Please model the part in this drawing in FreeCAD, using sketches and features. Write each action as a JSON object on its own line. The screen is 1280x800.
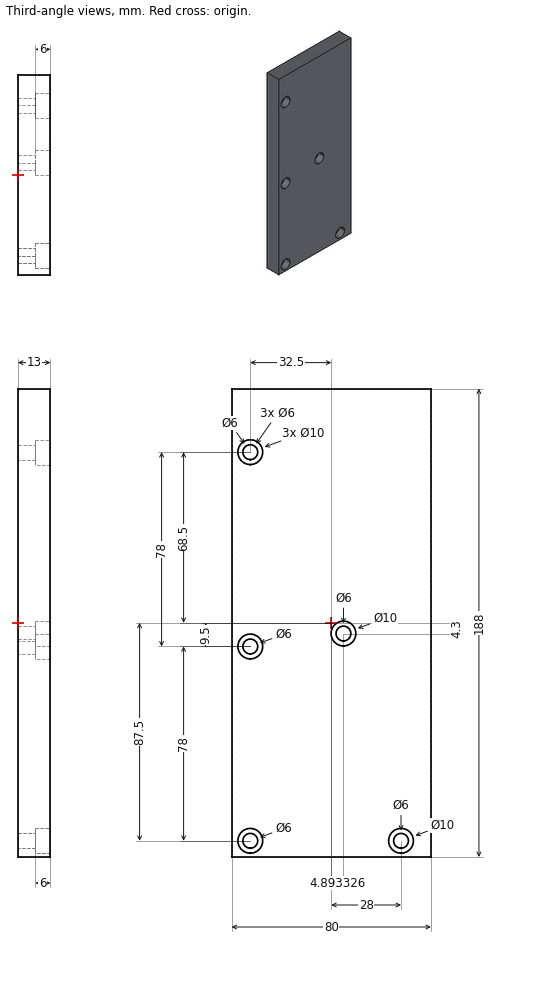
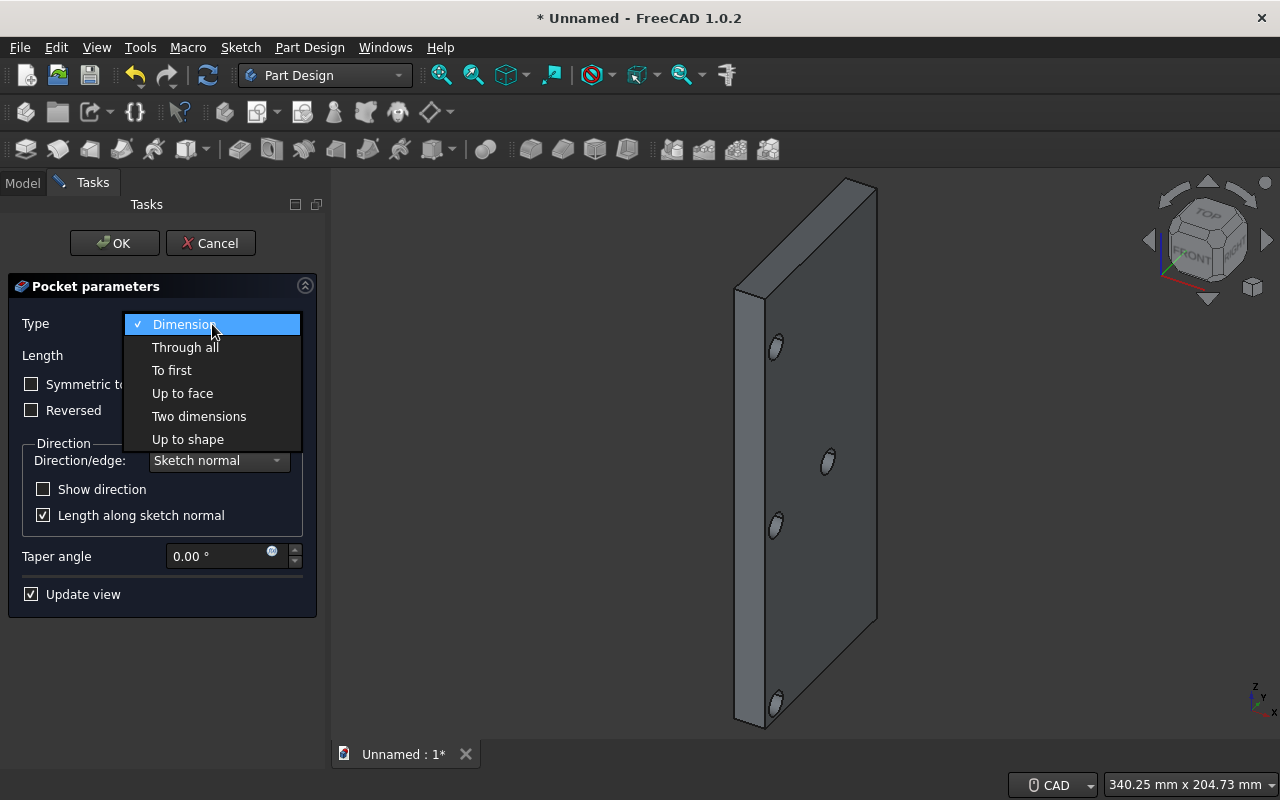
{"action": "left_click", "coordinate": [212, 370]}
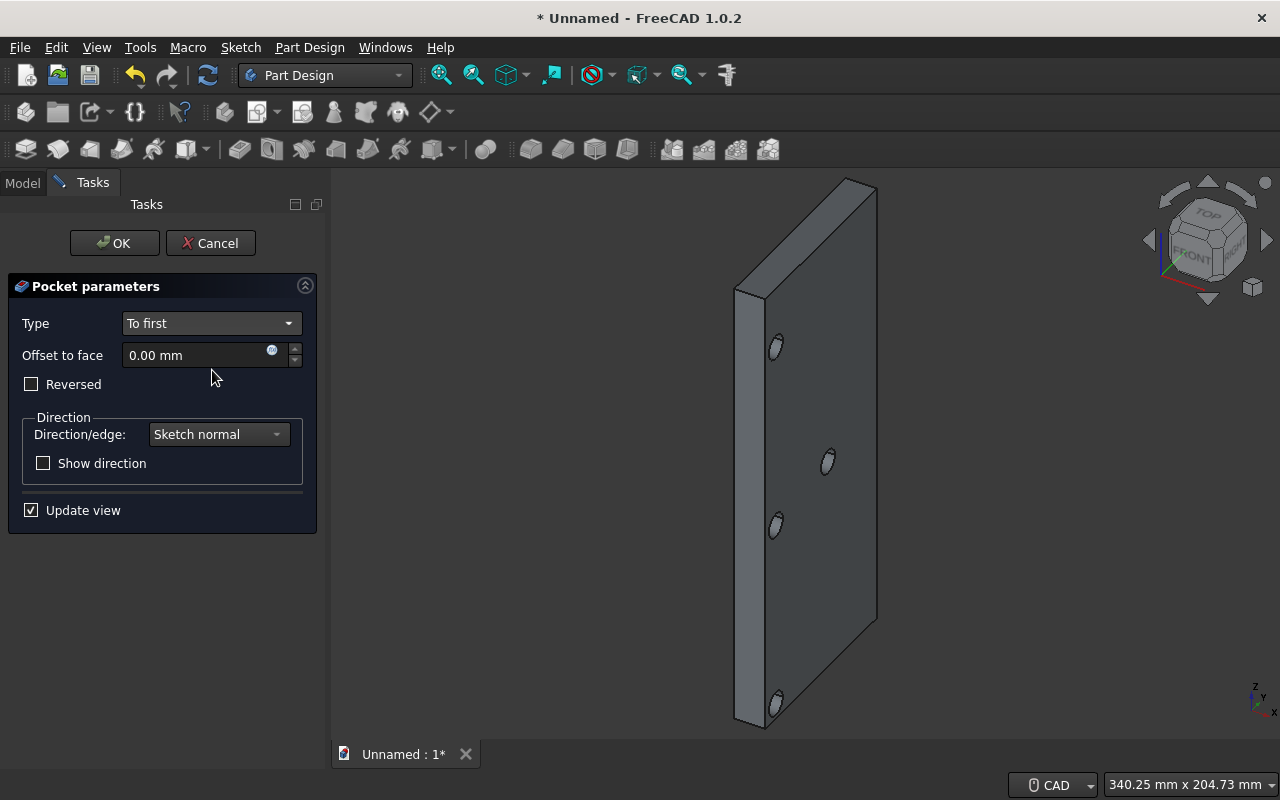
{"action": "left_click", "coordinate": [115, 243]}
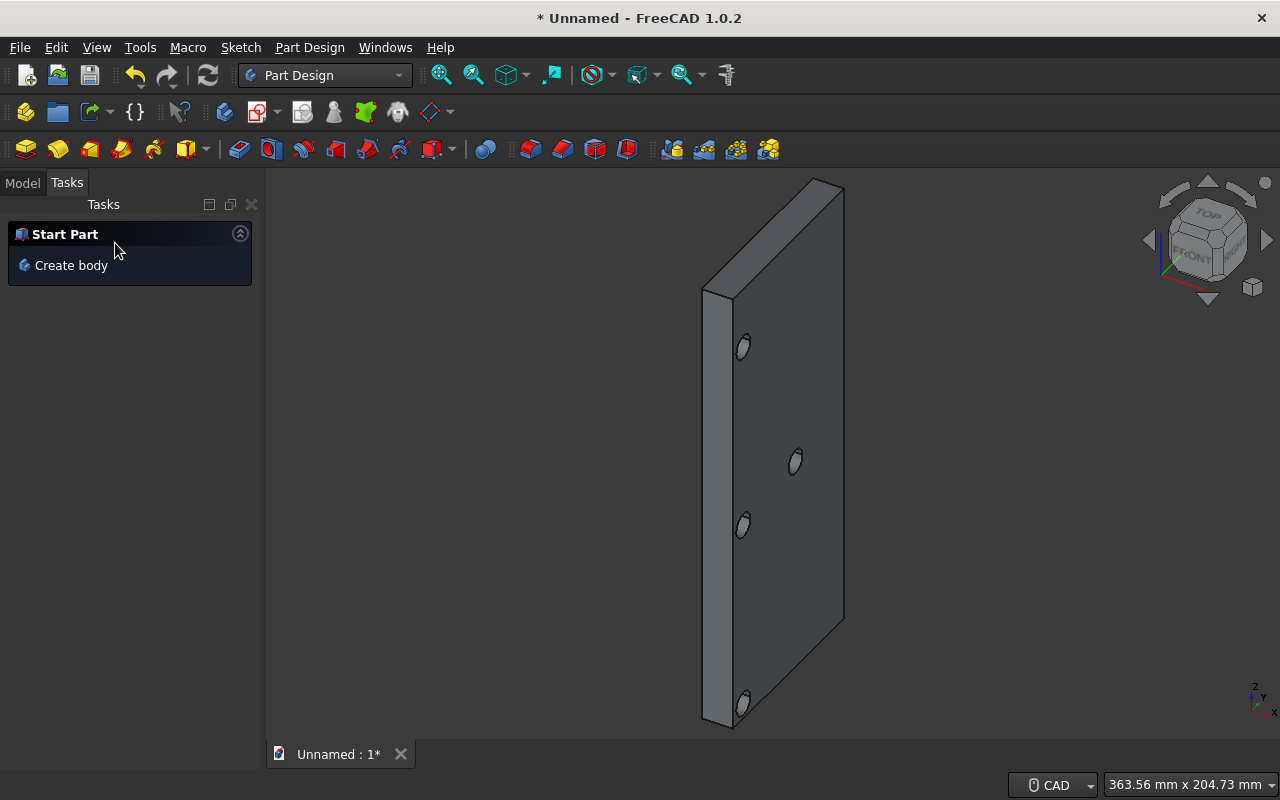
{"action": "left_click", "coordinate": [789, 580]}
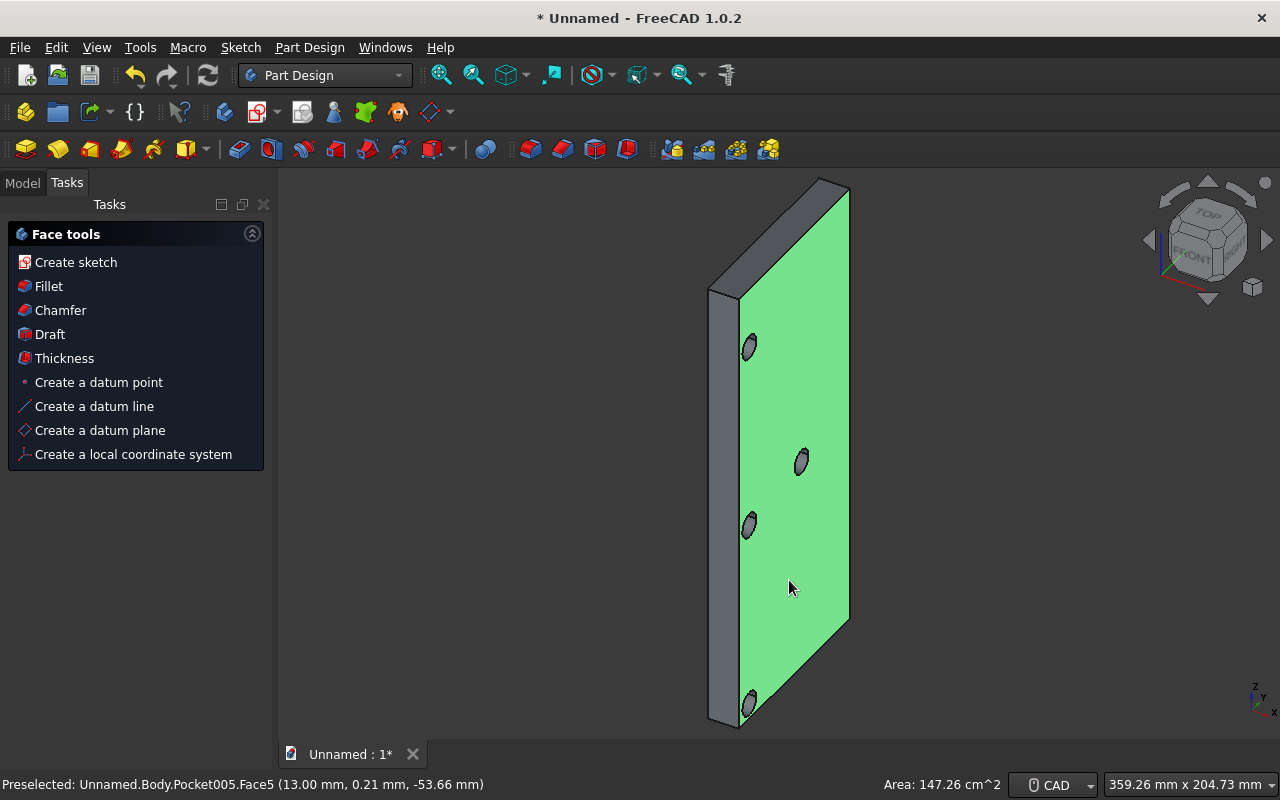
{"action": "left_click", "coordinate": [258, 112]}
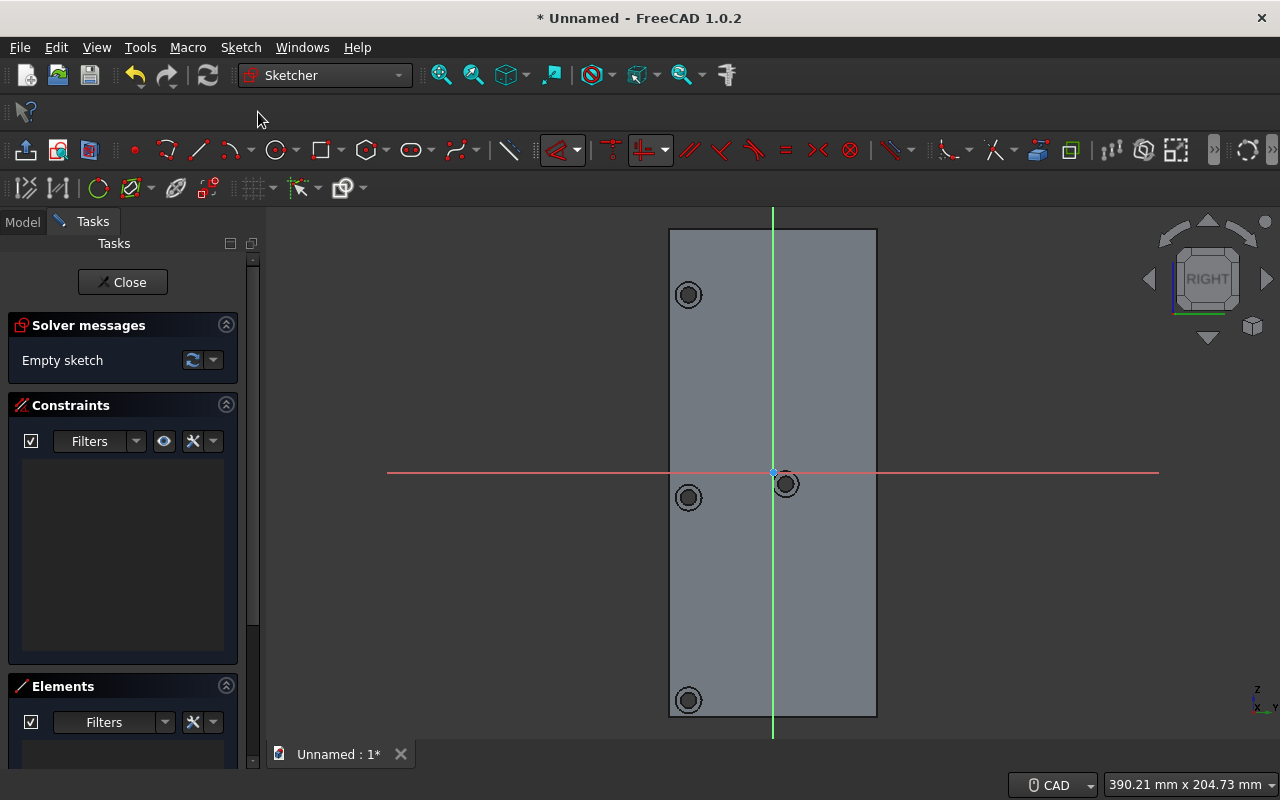
{"action": "scroll", "coordinate": [704, 473], "scroll_direction": "down", "scroll_amount": 5}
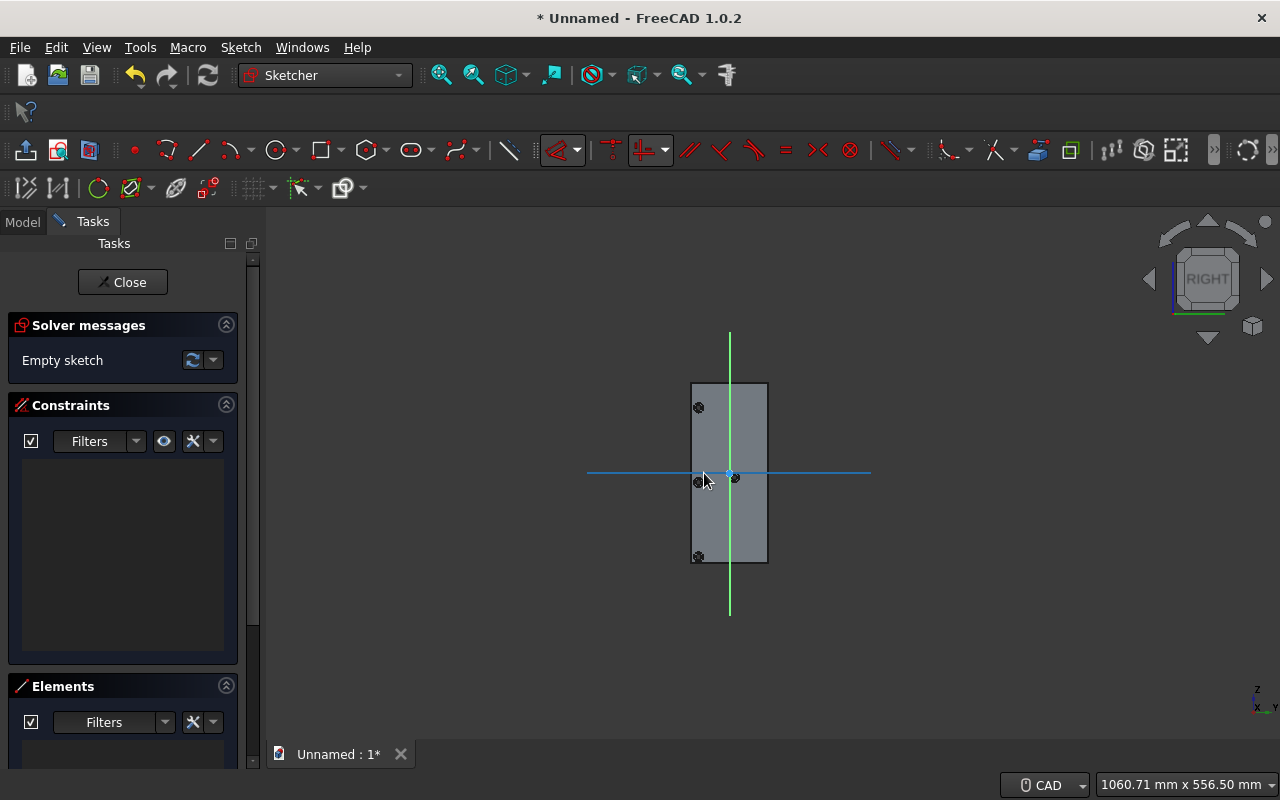
{"action": "scroll", "coordinate": [759, 561], "scroll_direction": "up", "scroll_amount": 15}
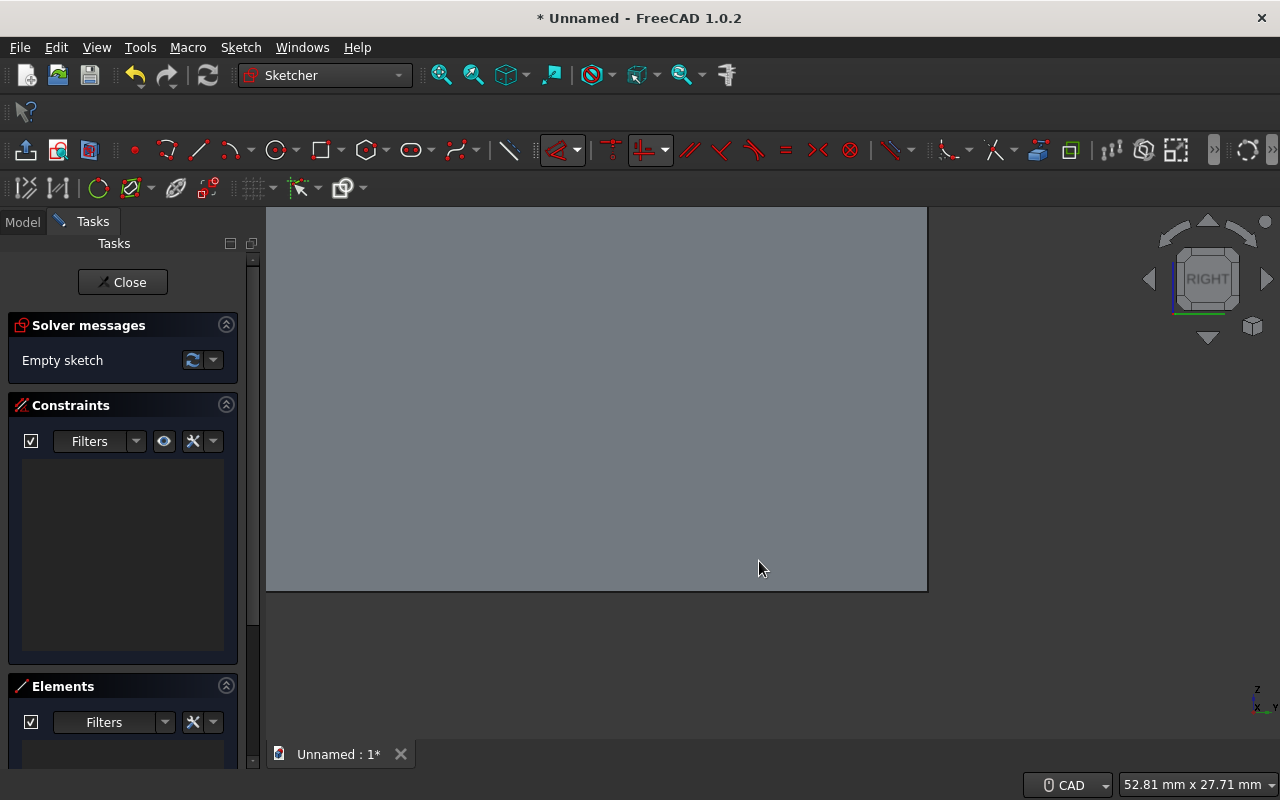
{"action": "scroll", "coordinate": [690, 460], "scroll_direction": "up", "scroll_amount": 3}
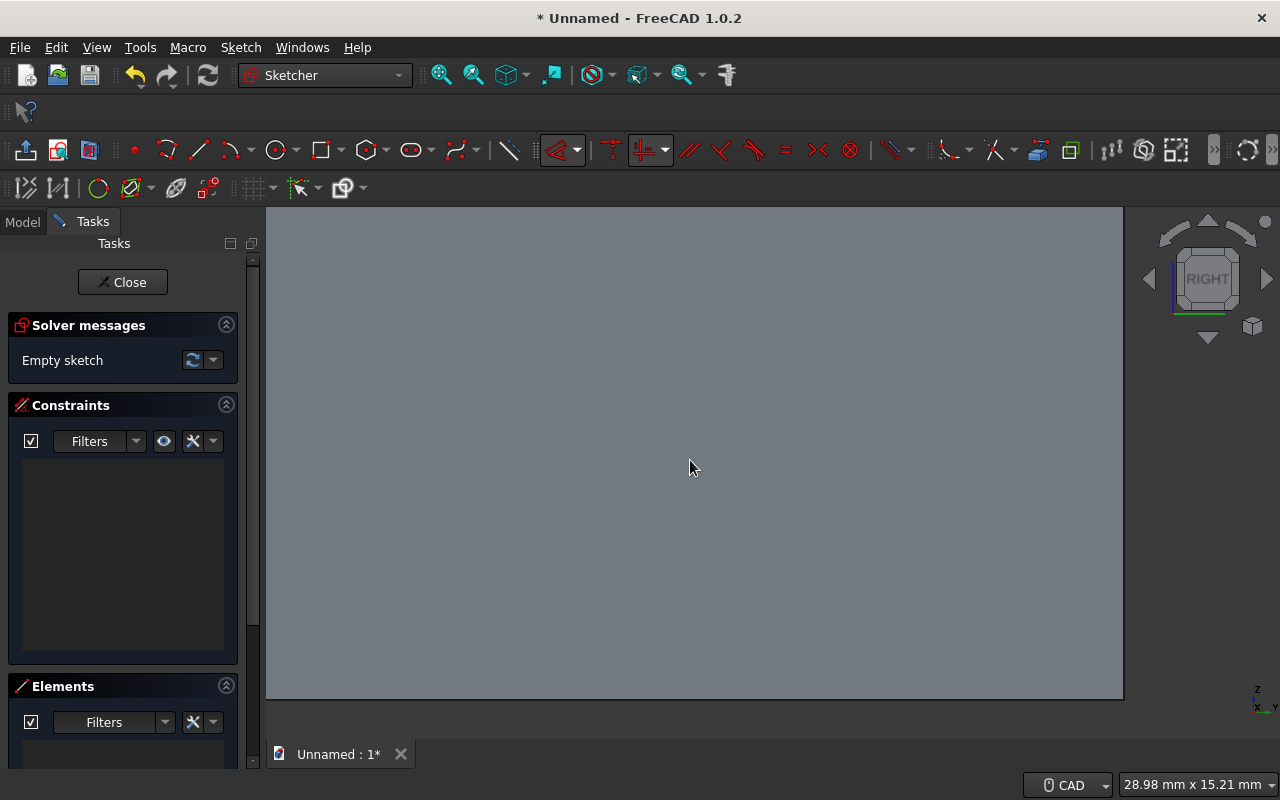
{"action": "left_click", "coordinate": [276, 150]}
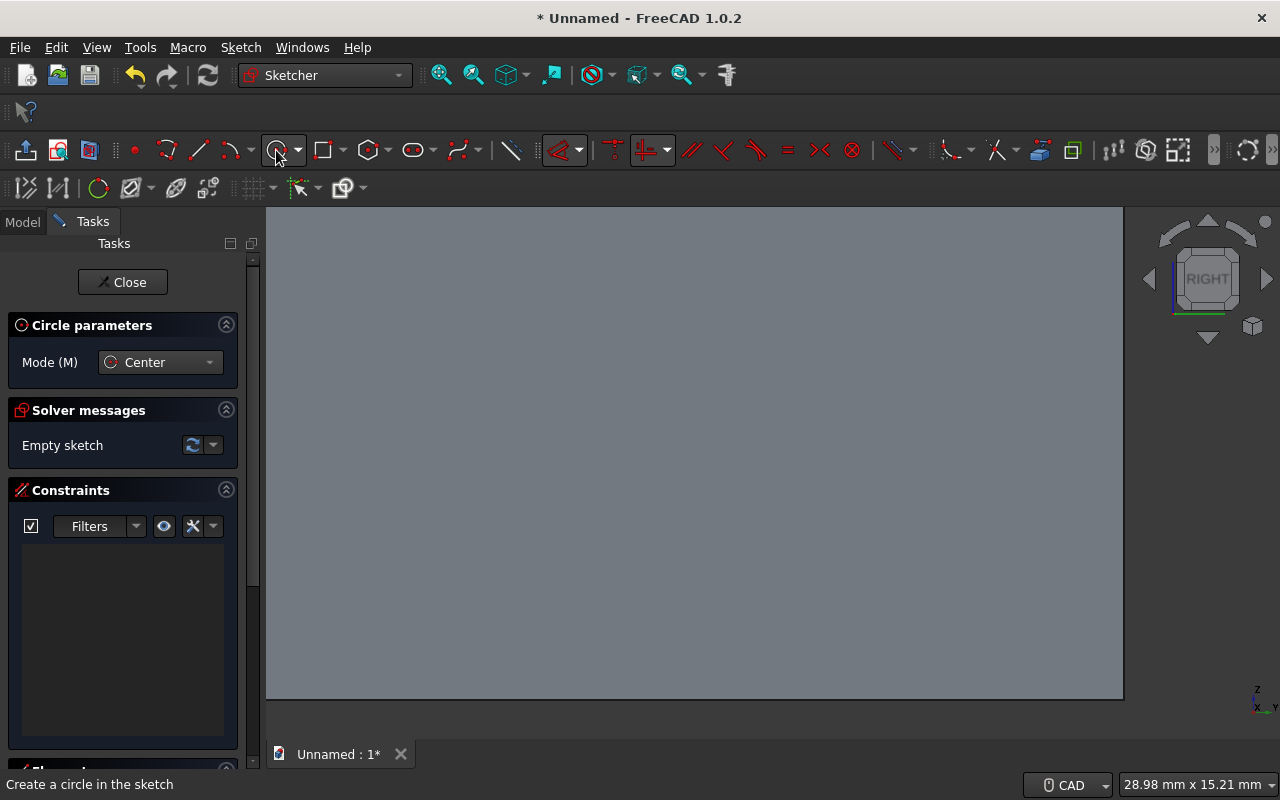
{"action": "left_click", "coordinate": [704, 473]}
{"action": "left_click", "coordinate": [828, 349]}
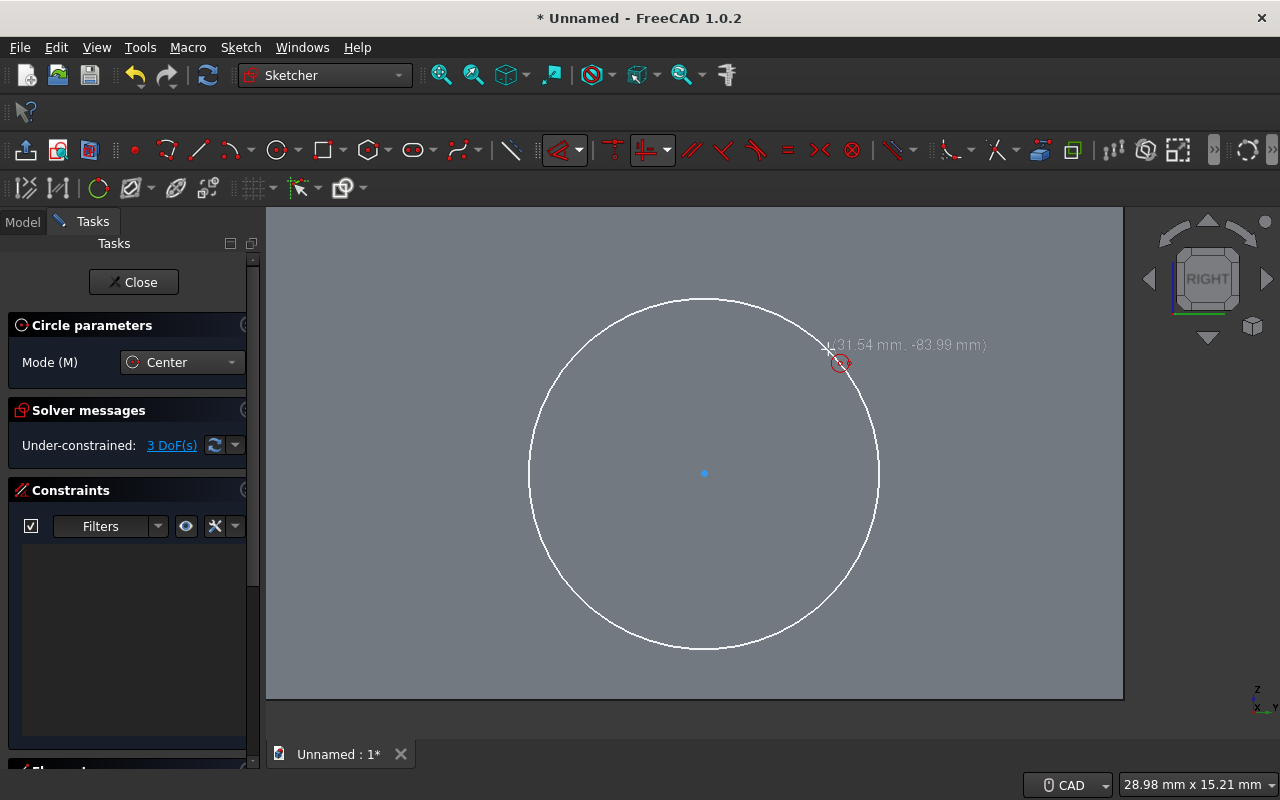
{"action": "left_click", "coordinate": [704, 474]}
{"action": "left_click", "coordinate": [778, 399]}
{"action": "key", "text": "Escape"}